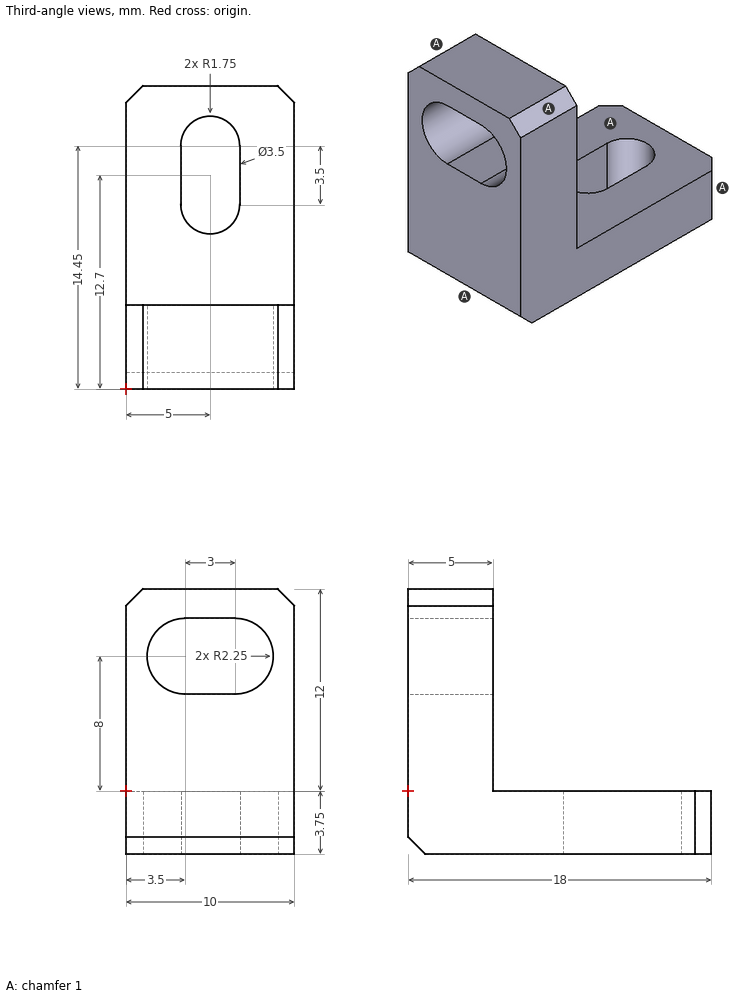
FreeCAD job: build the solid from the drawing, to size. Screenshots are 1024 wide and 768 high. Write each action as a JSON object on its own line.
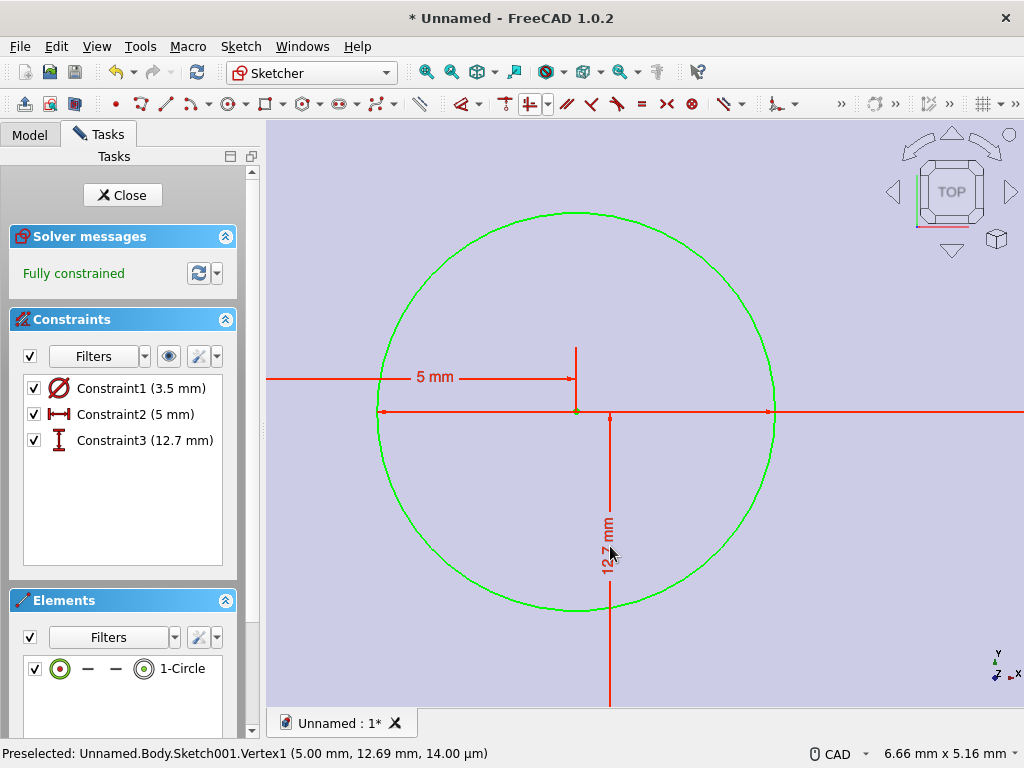
{"action": "left_click", "coordinate": [123, 195]}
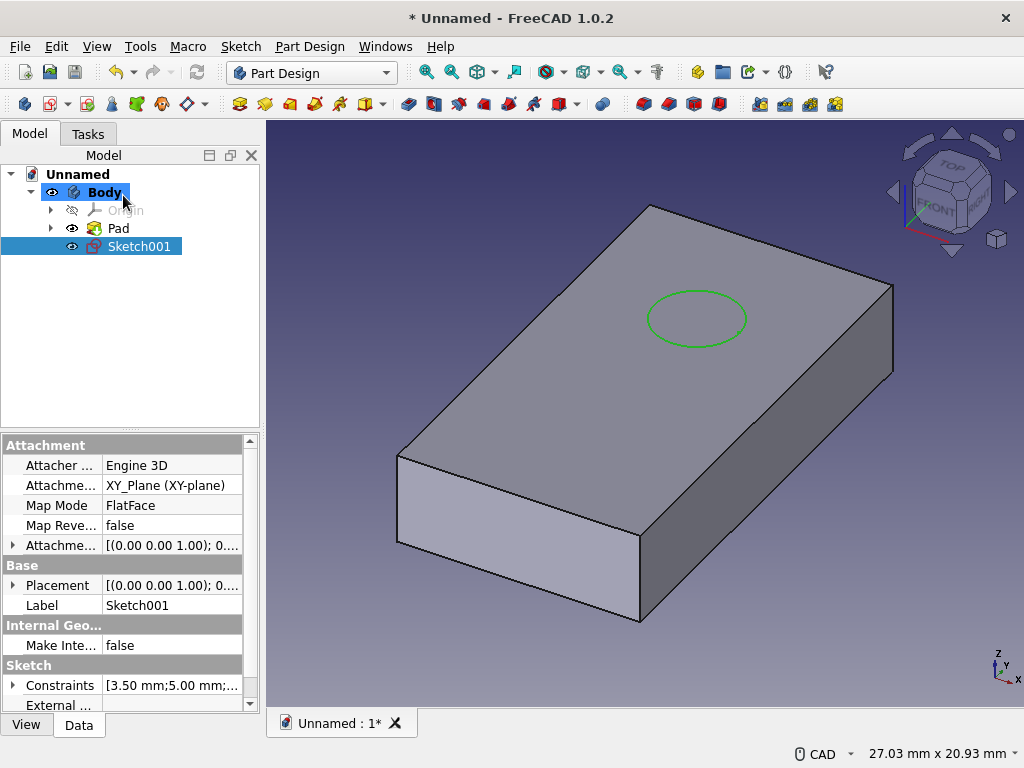
{"action": "left_click", "coordinate": [409, 104]}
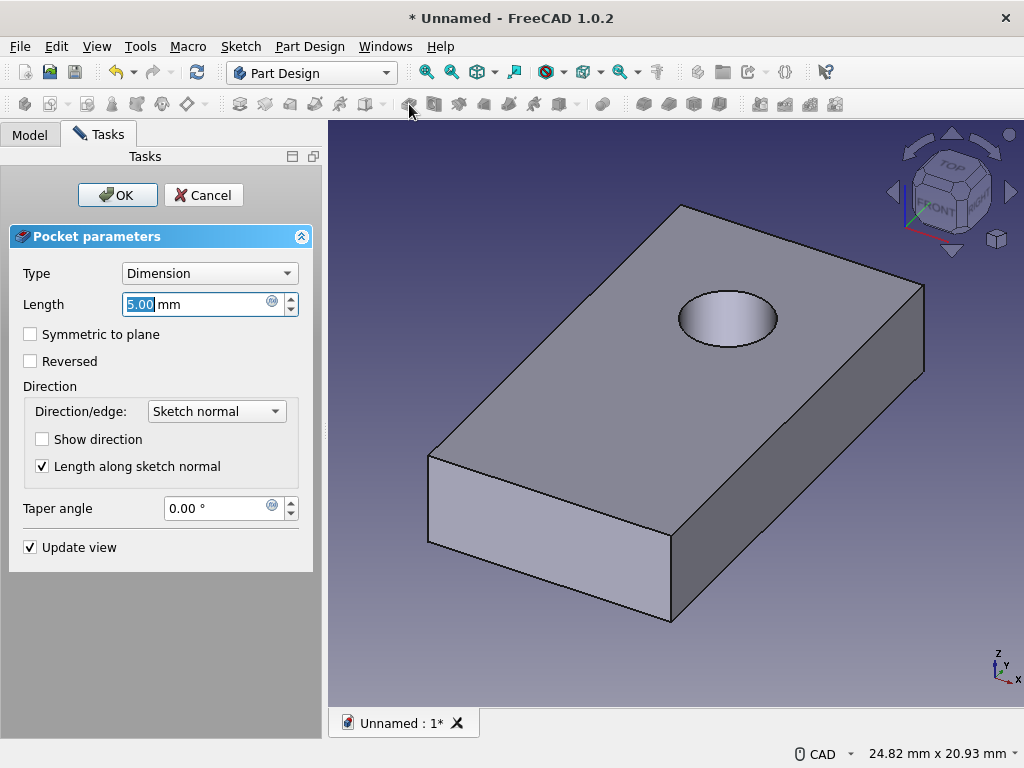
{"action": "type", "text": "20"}
{"action": "key", "text": "Tab"}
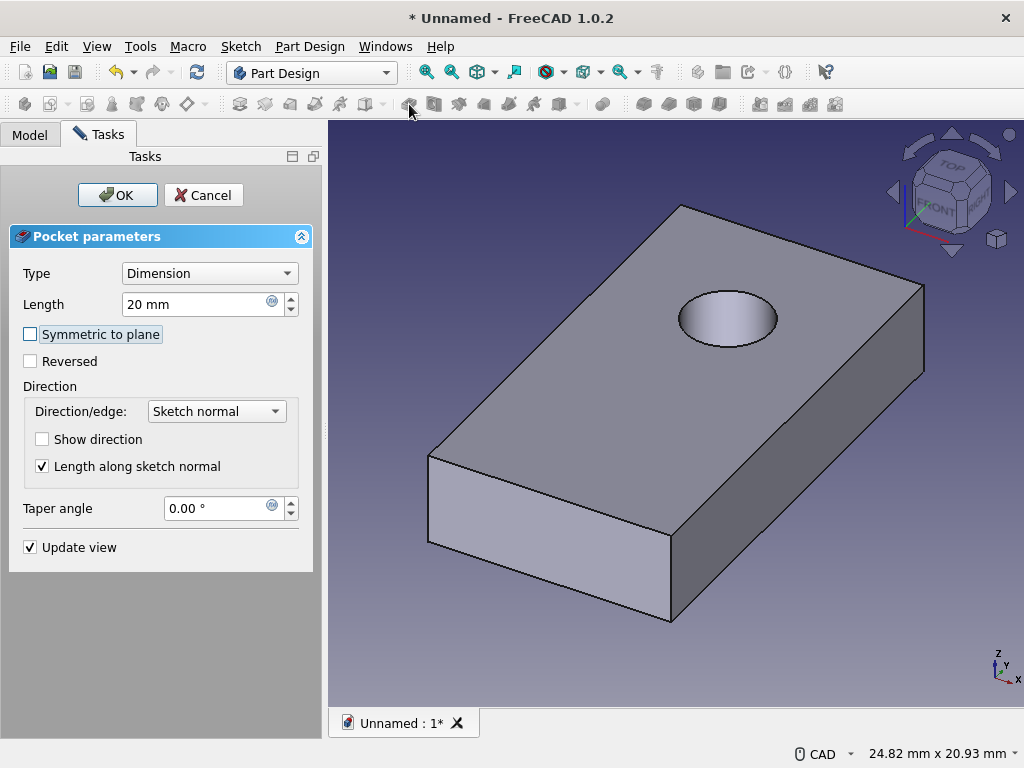
{"action": "left_click", "coordinate": [118, 195]}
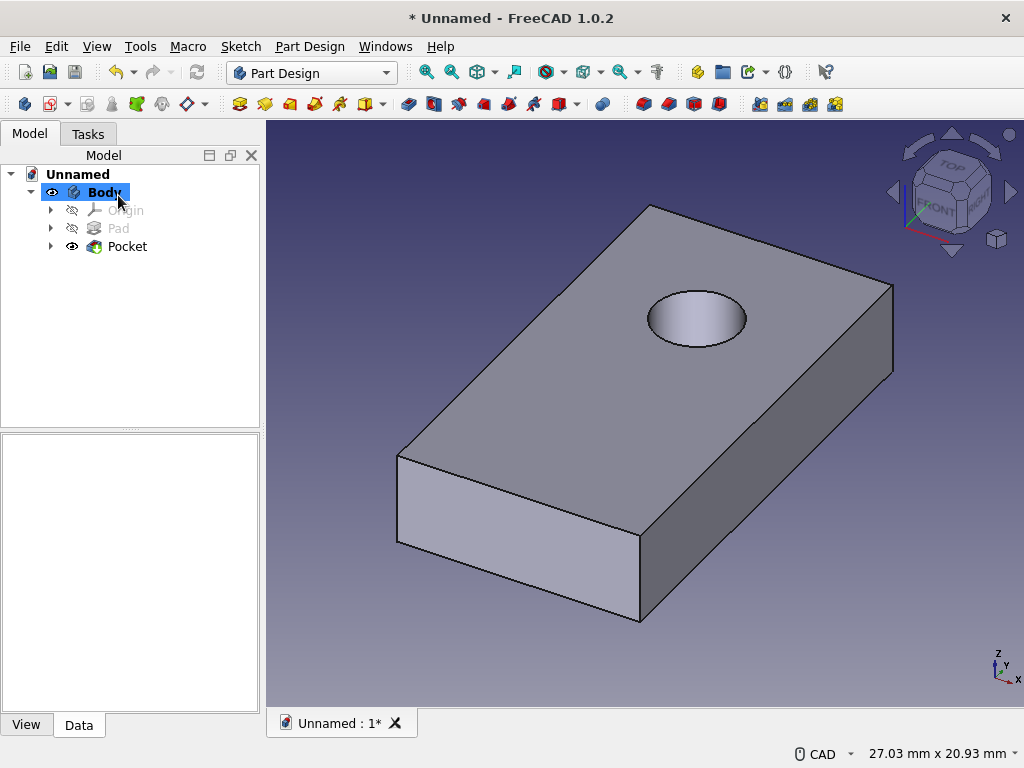
{"action": "left_click", "coordinate": [50, 104]}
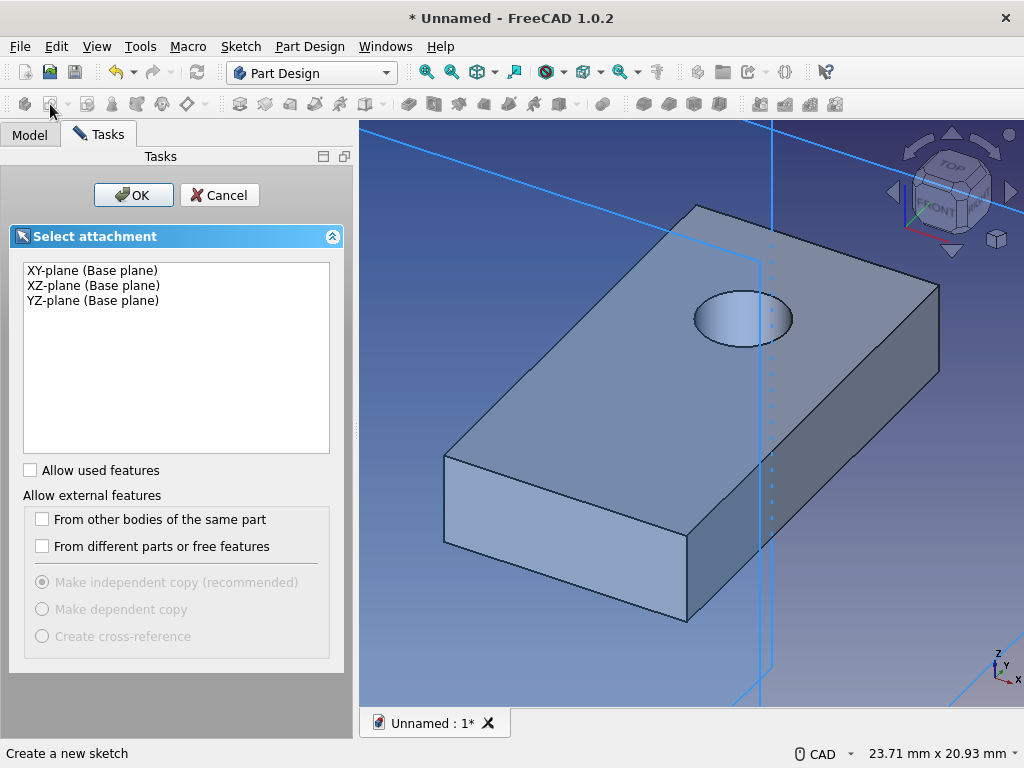
{"action": "left_click", "coordinate": [84, 286]}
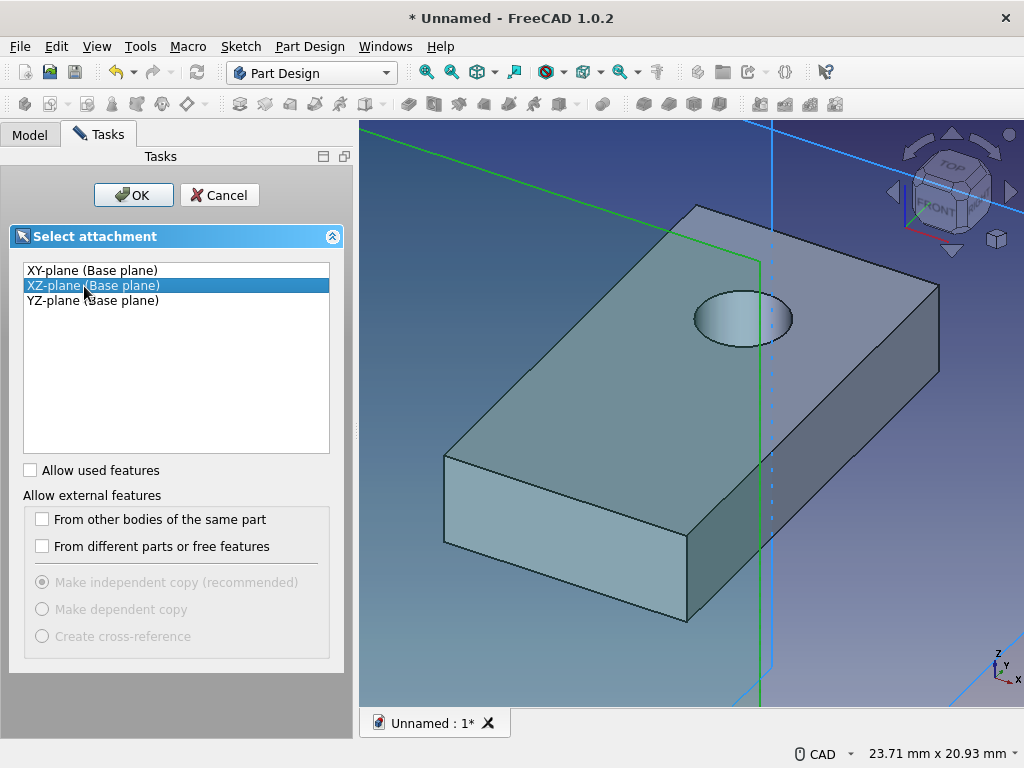
{"action": "left_click", "coordinate": [134, 195]}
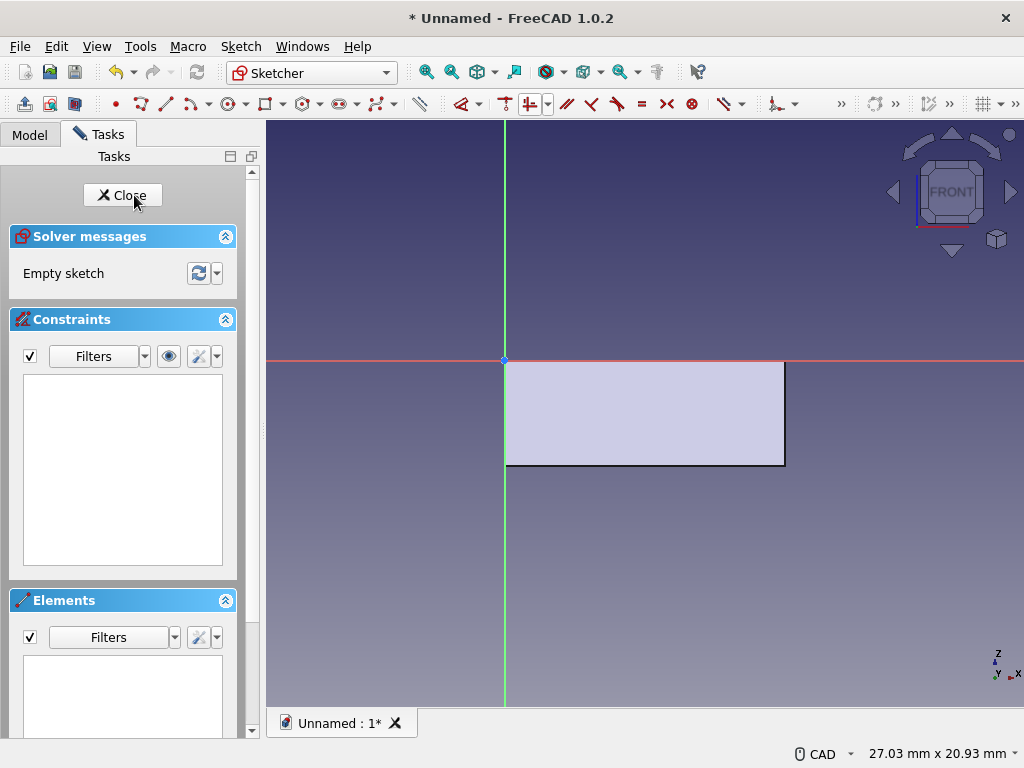
{"action": "scroll", "coordinate": [437, 679], "scroll_direction": "down", "scroll_amount": 2}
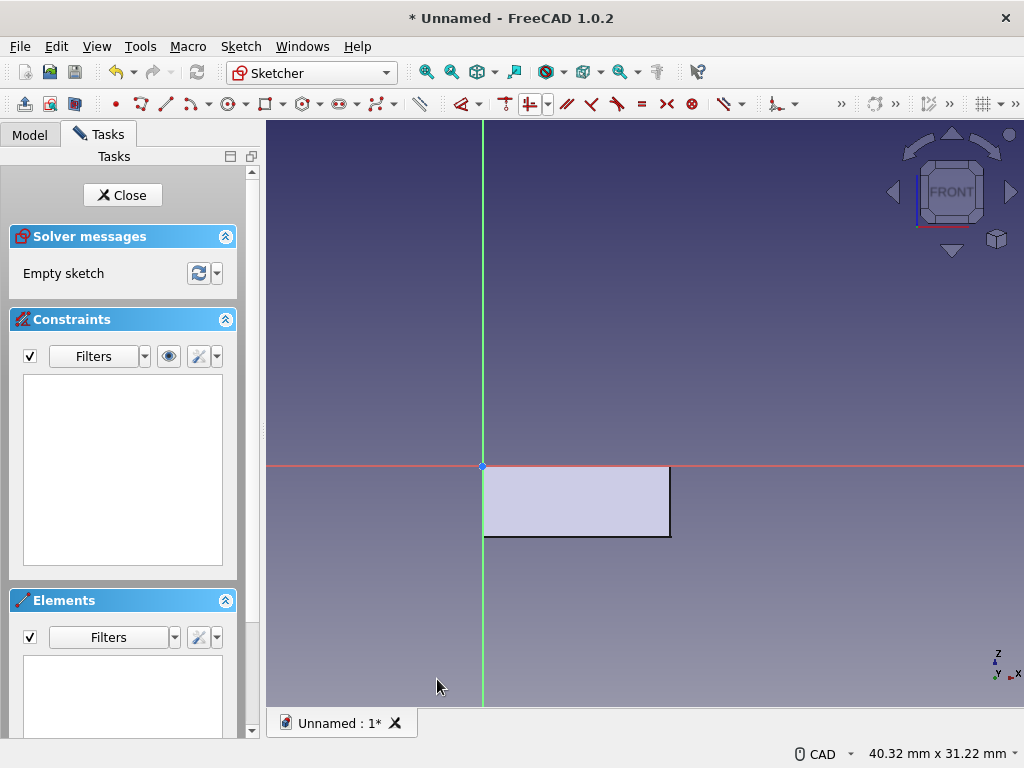
{"action": "scroll", "coordinate": [577, 280], "scroll_direction": "up", "scroll_amount": 3}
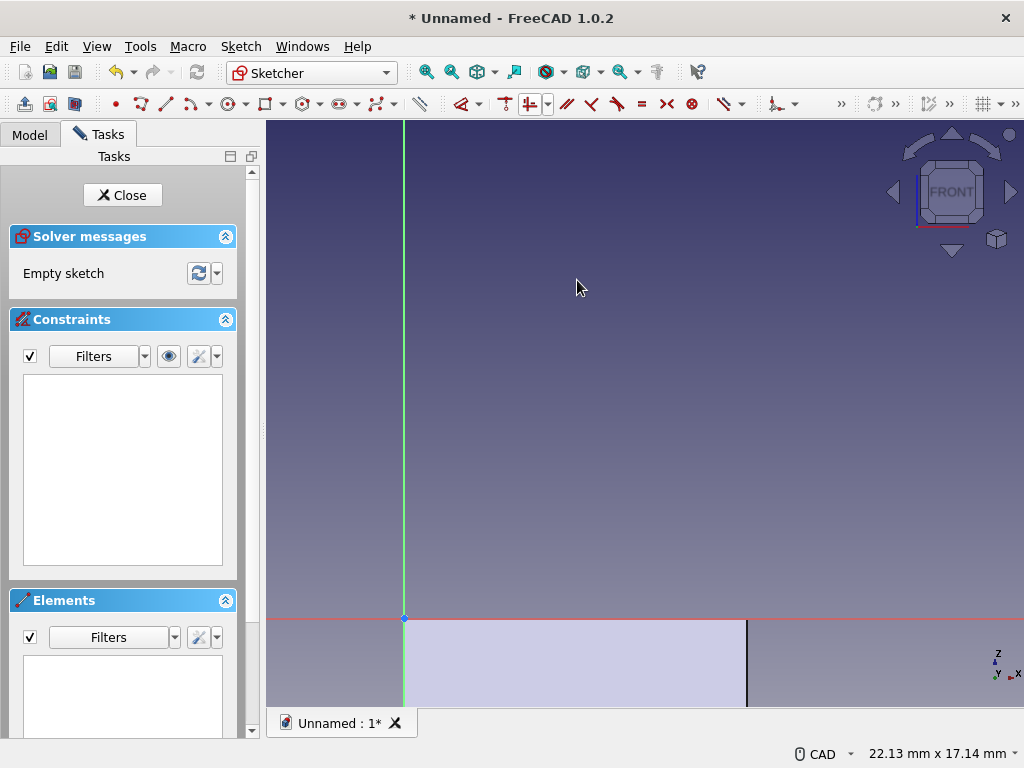
{"action": "left_click", "coordinate": [264, 104]}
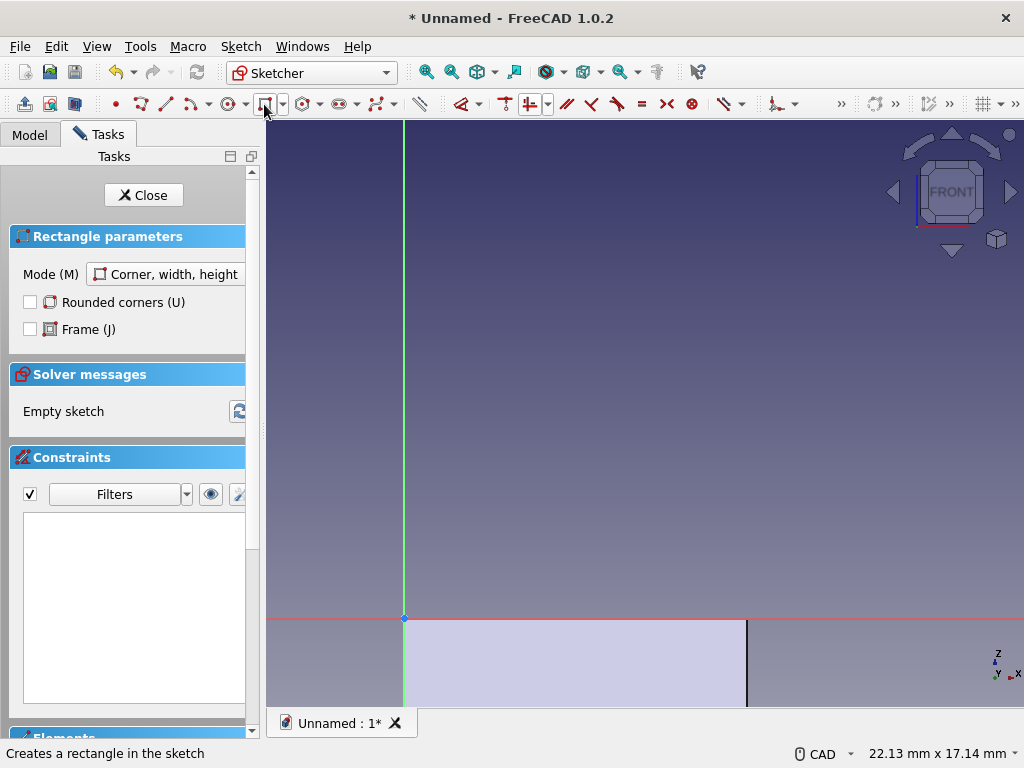
{"action": "left_click", "coordinate": [404, 619]}
{"action": "mouse_move", "coordinate": [747, 208]}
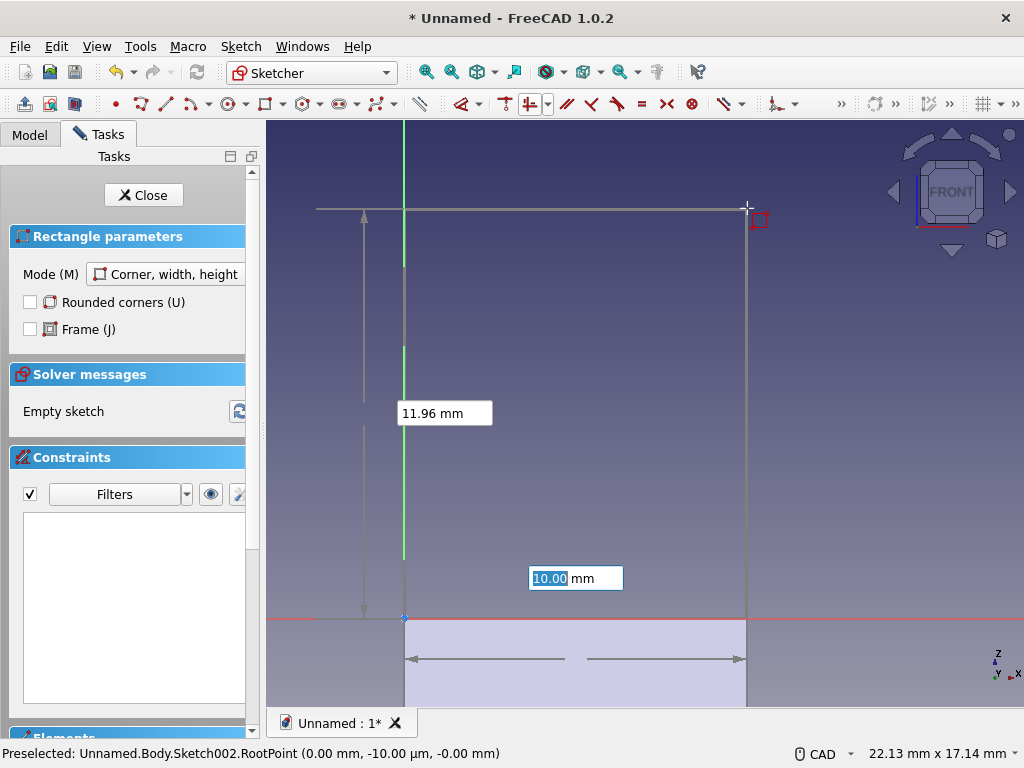
{"action": "type", "text": "10"}
{"action": "key", "text": "Tab"}
{"action": "type", "text": "12"}
{"action": "key", "text": "Return"}
{"action": "key", "text": "Escape"}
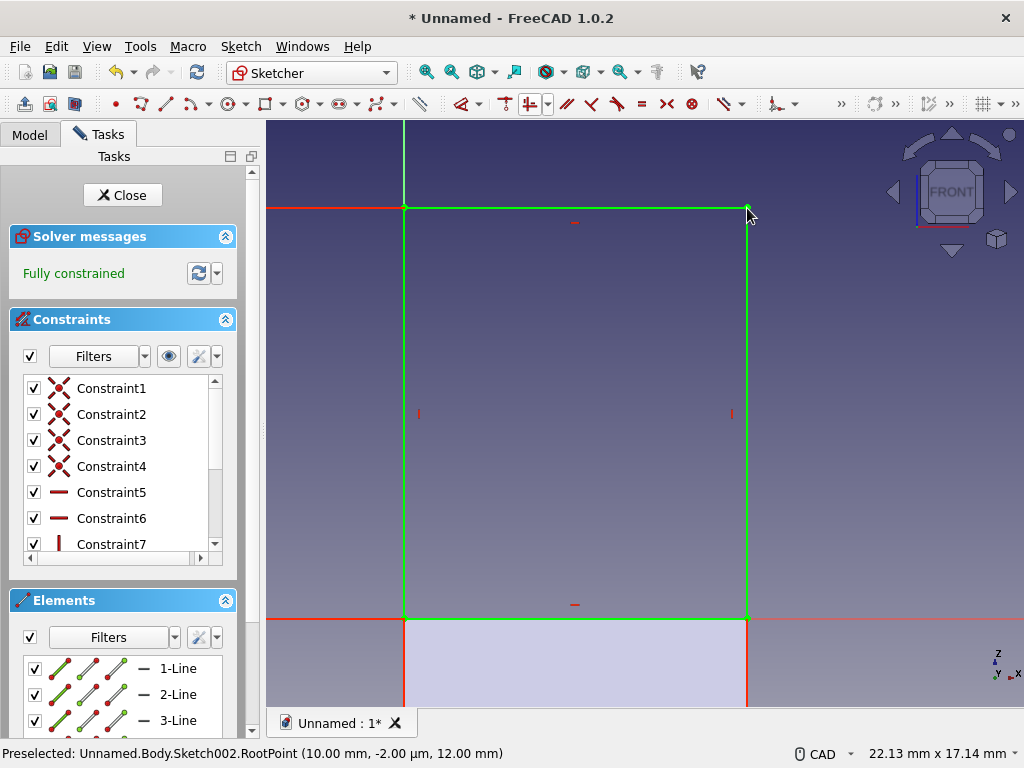
{"action": "left_click", "coordinate": [123, 195]}